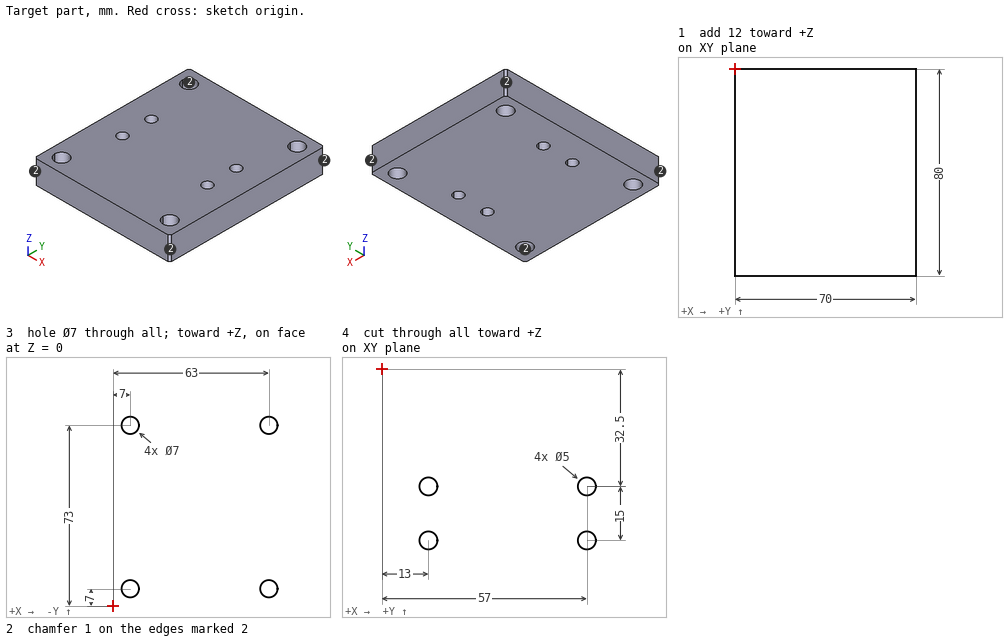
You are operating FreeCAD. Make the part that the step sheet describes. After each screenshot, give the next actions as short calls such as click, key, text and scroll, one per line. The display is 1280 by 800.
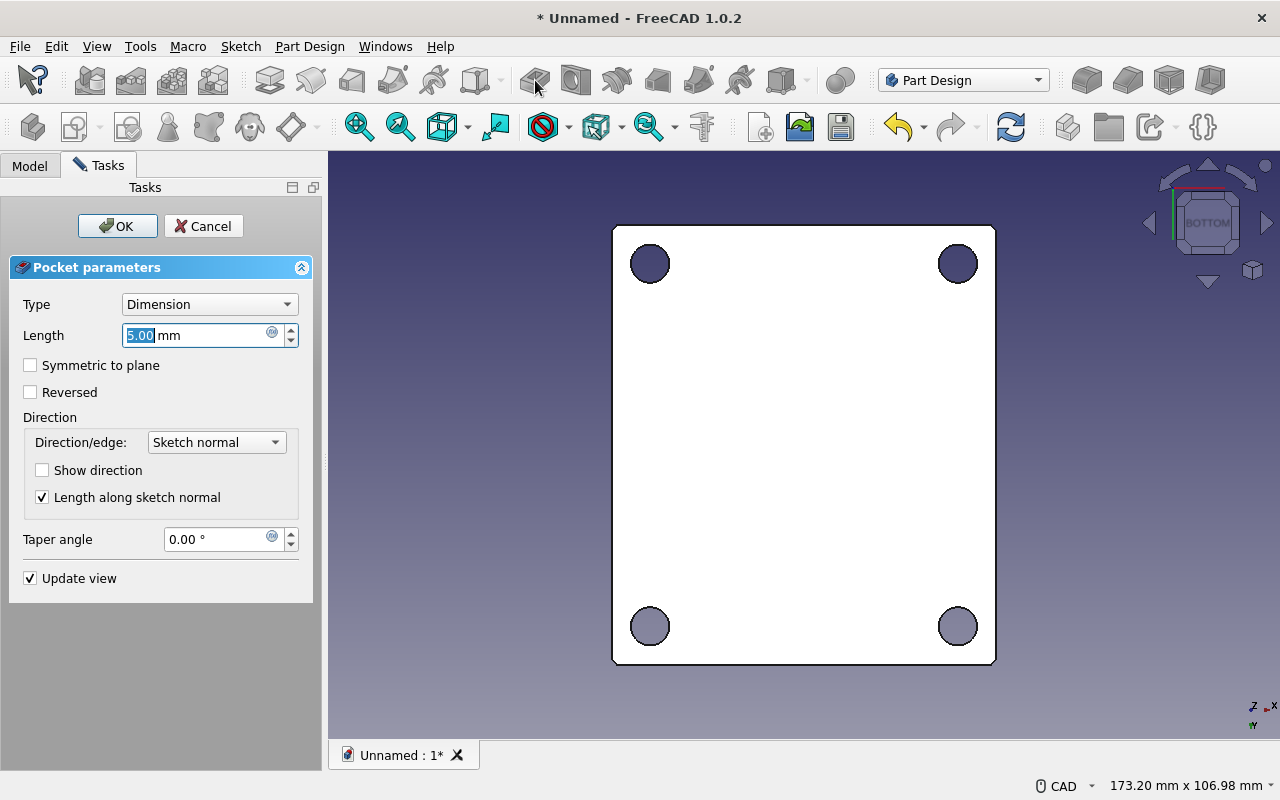
click(210, 304)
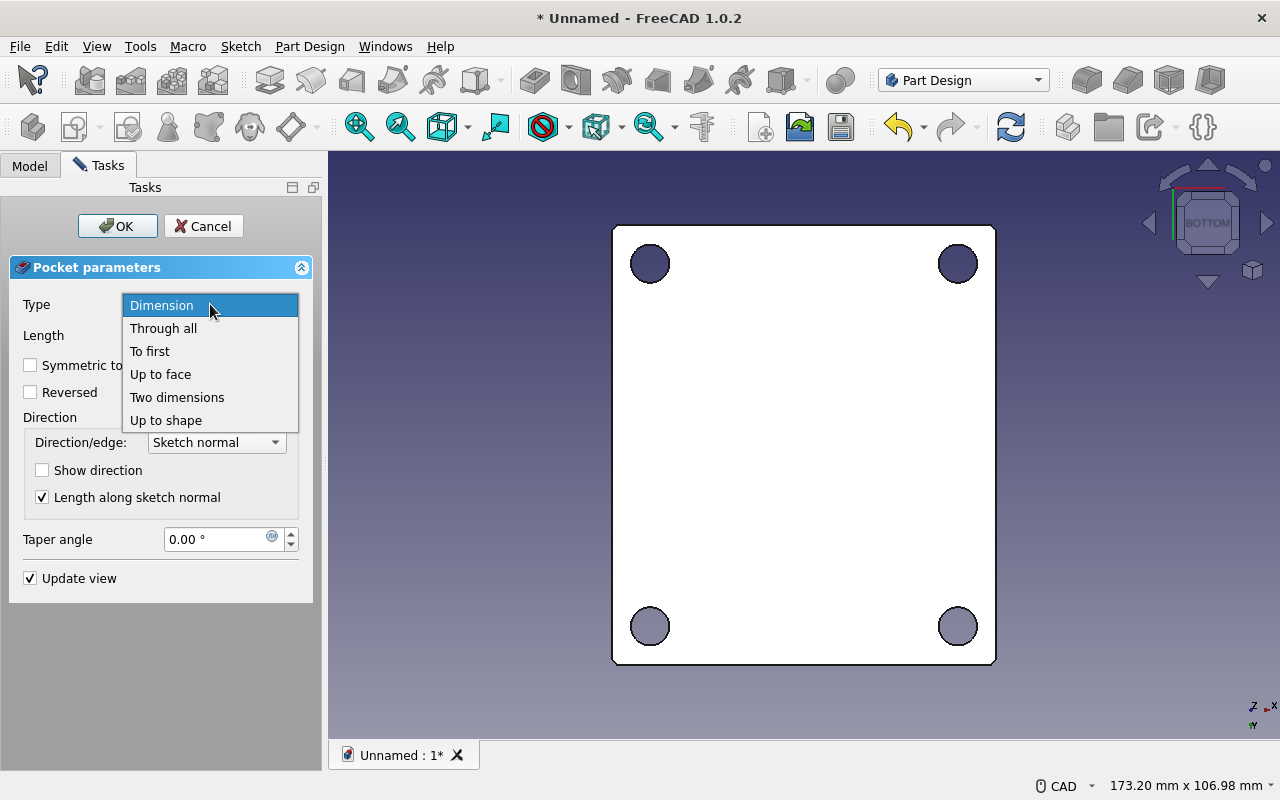
click(208, 328)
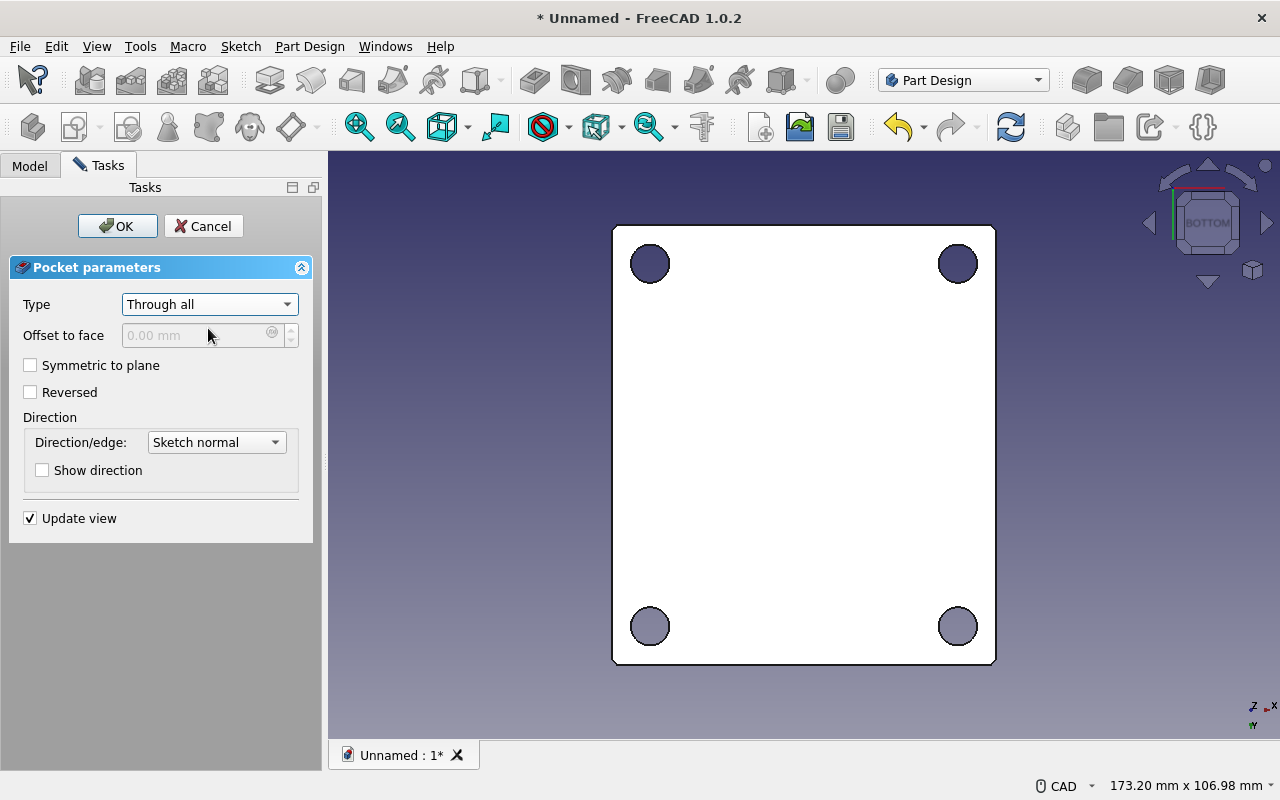
click(31, 392)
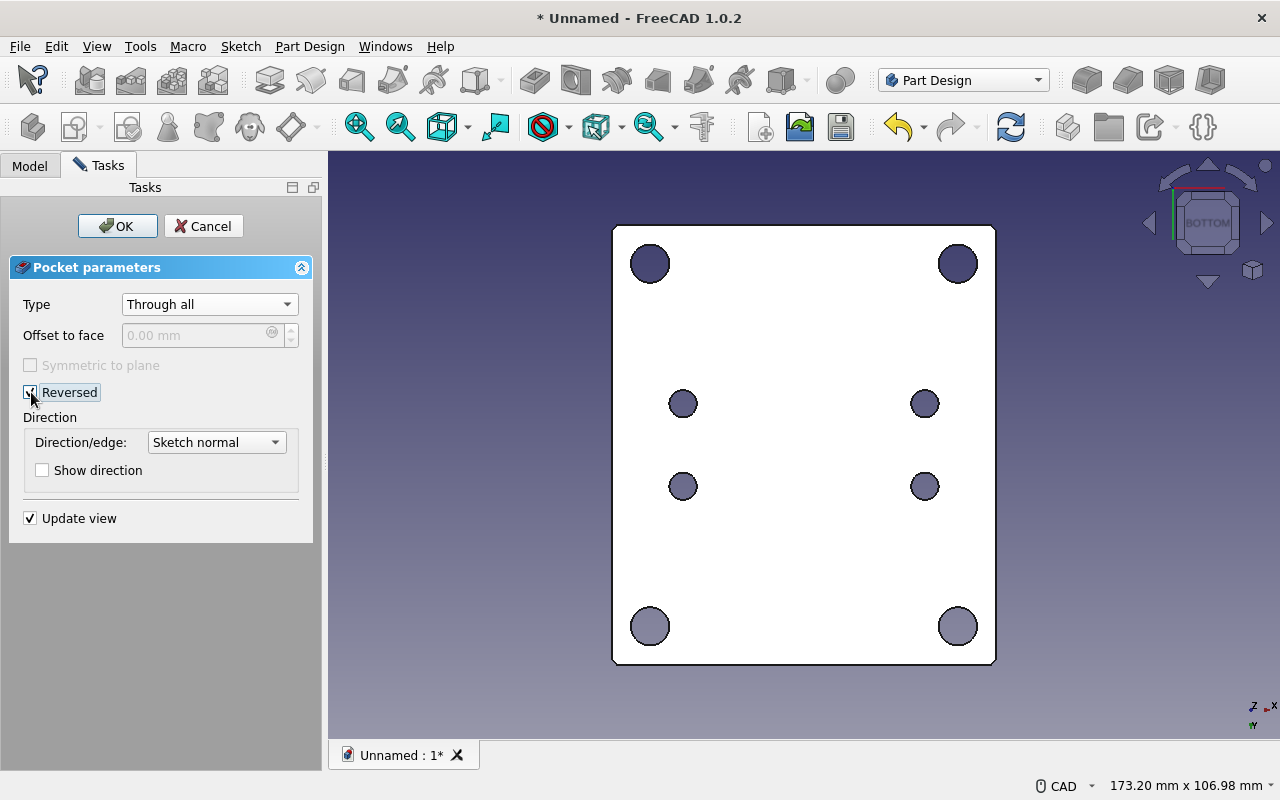
click(118, 226)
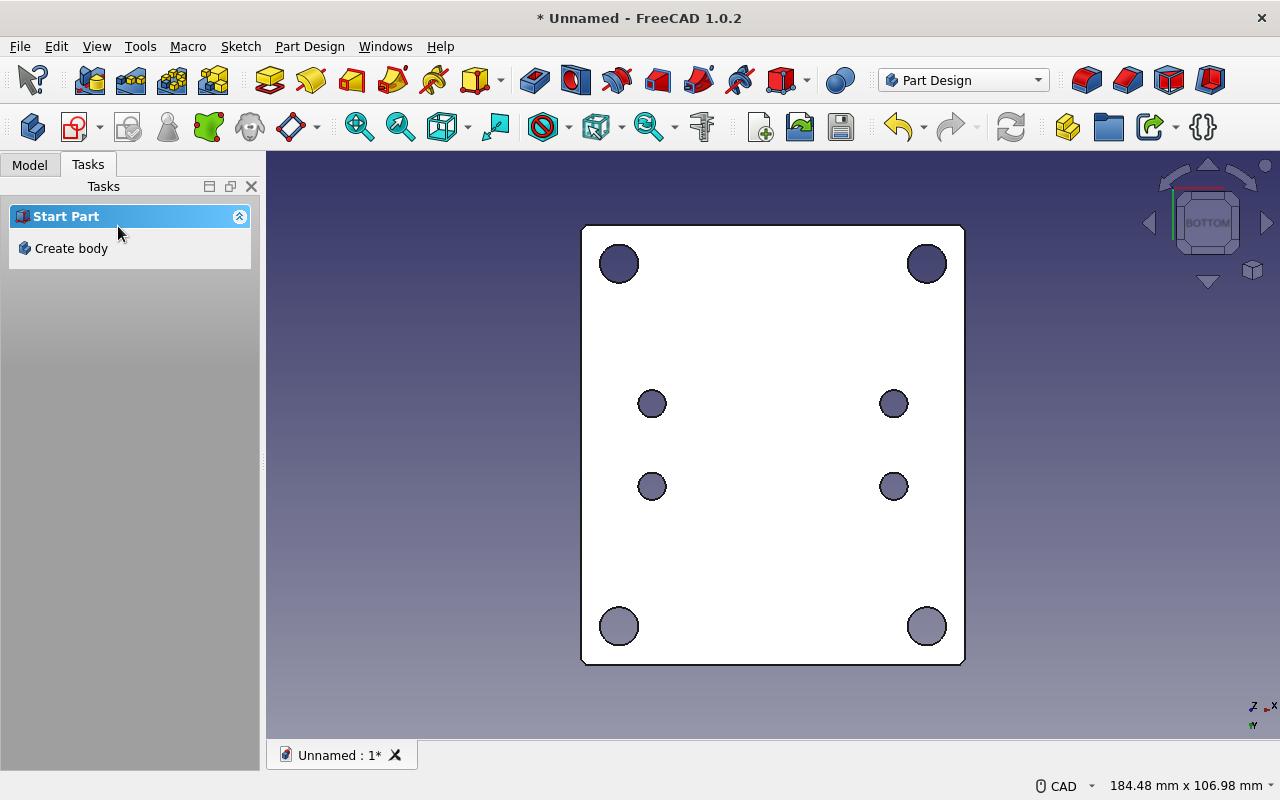
key(0)